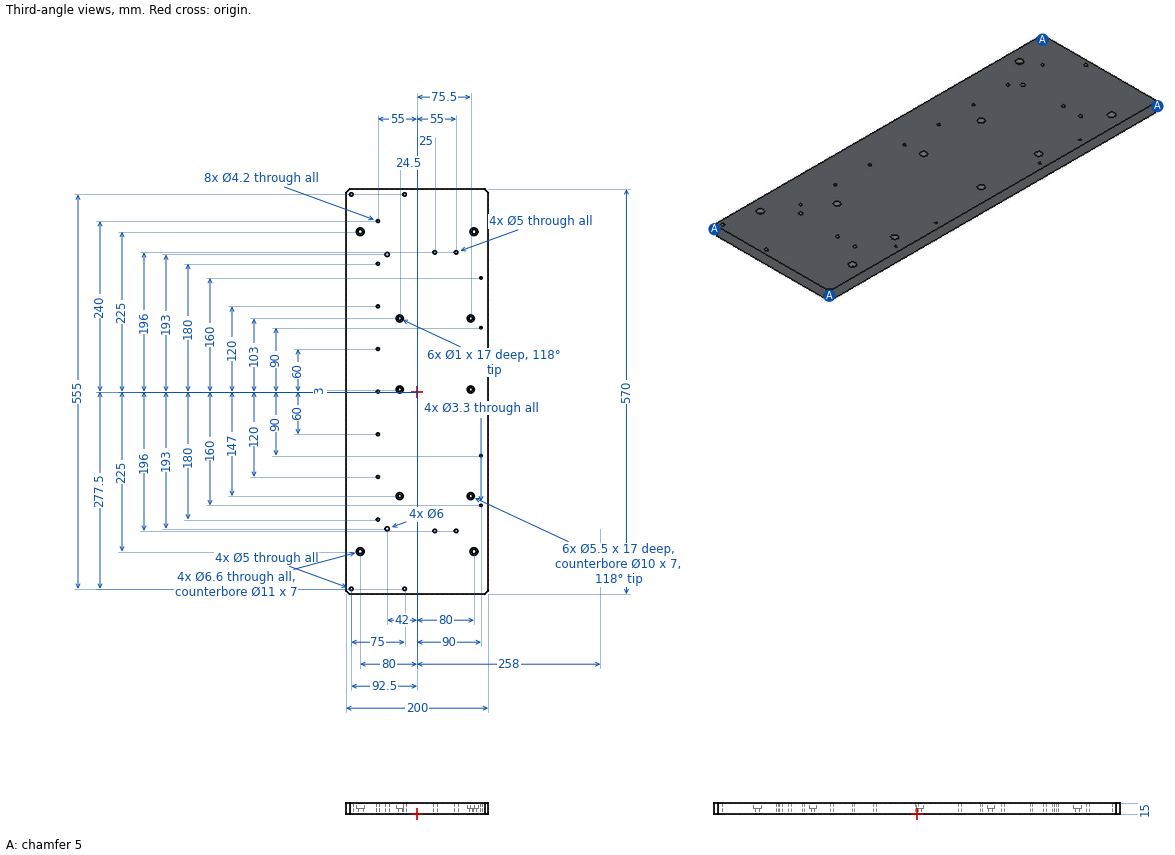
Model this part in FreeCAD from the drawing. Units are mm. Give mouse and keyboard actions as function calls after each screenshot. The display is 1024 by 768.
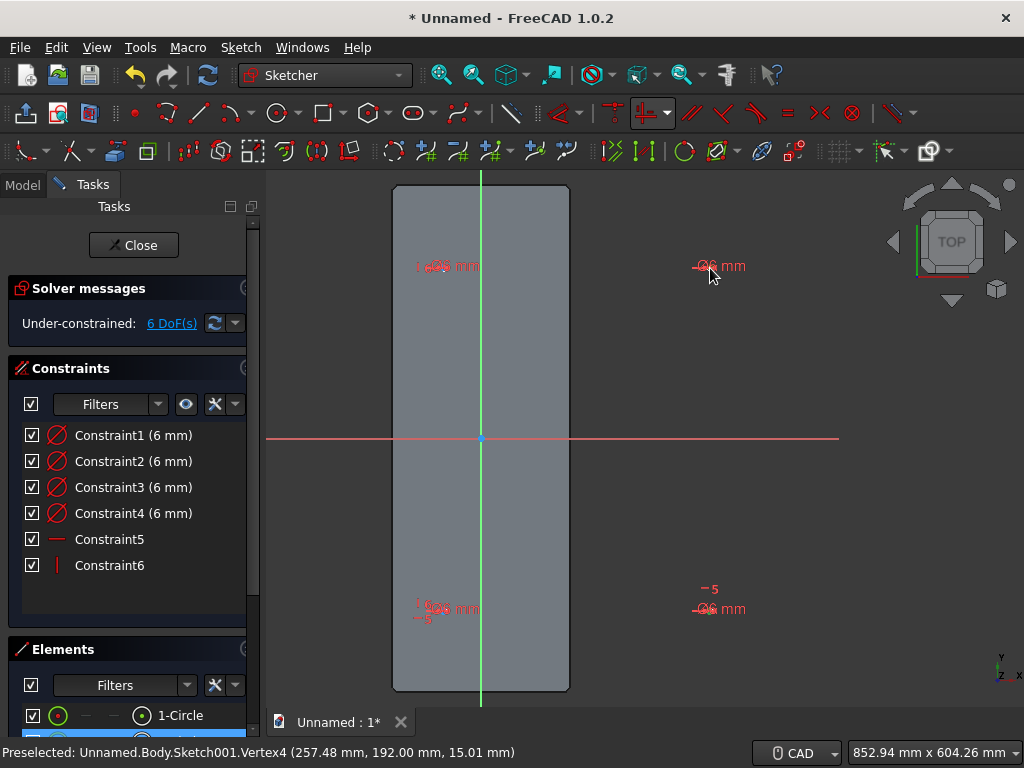
click(670, 114)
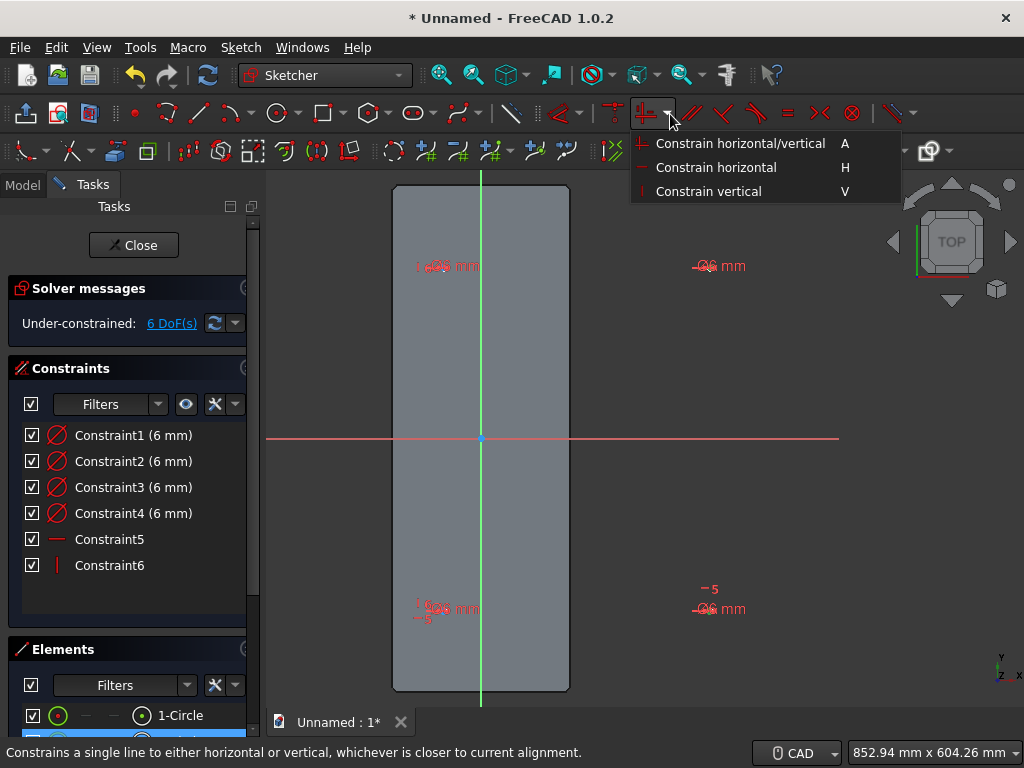
click(766, 191)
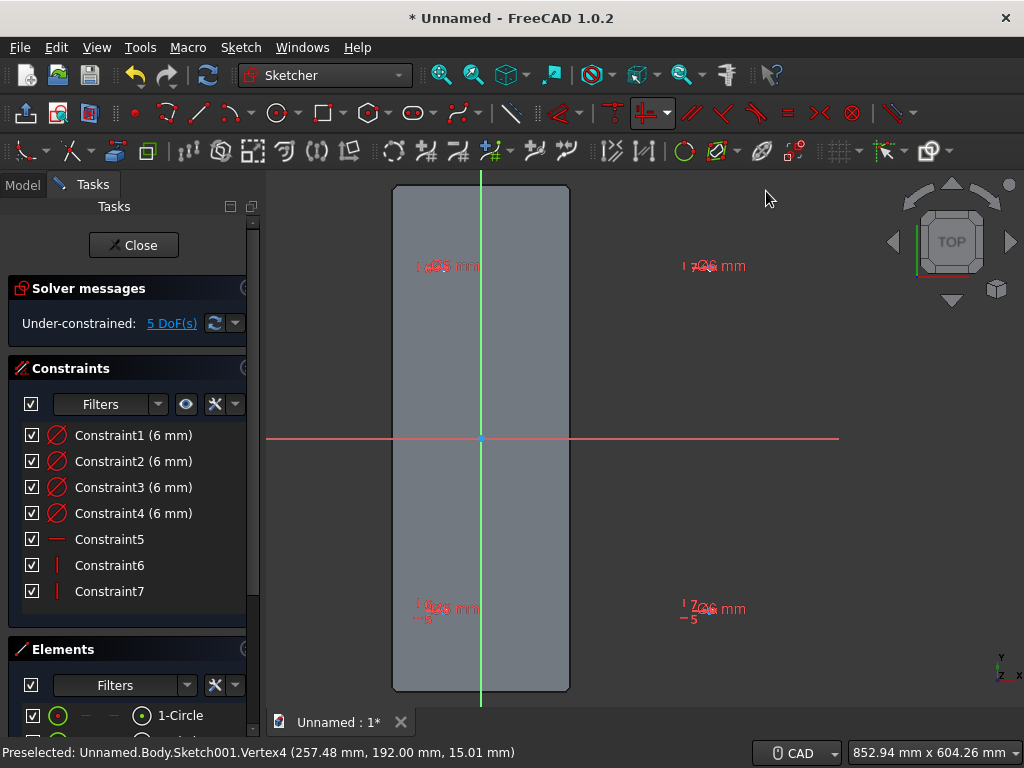
click(444, 268)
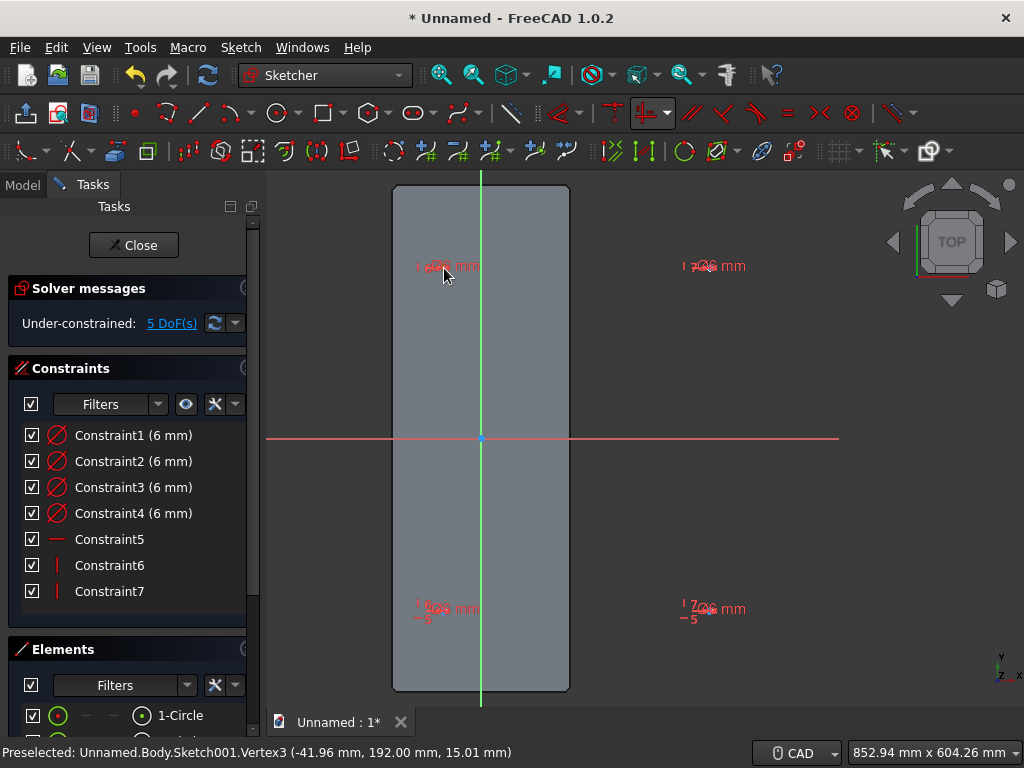
click(710, 268)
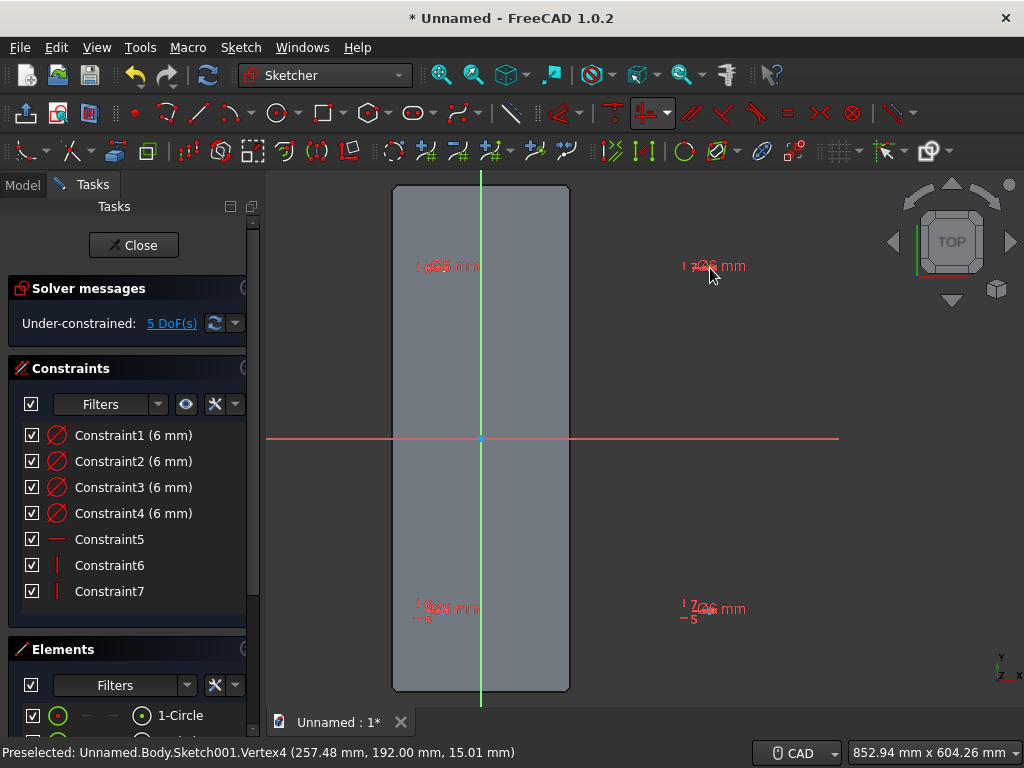
click(670, 114)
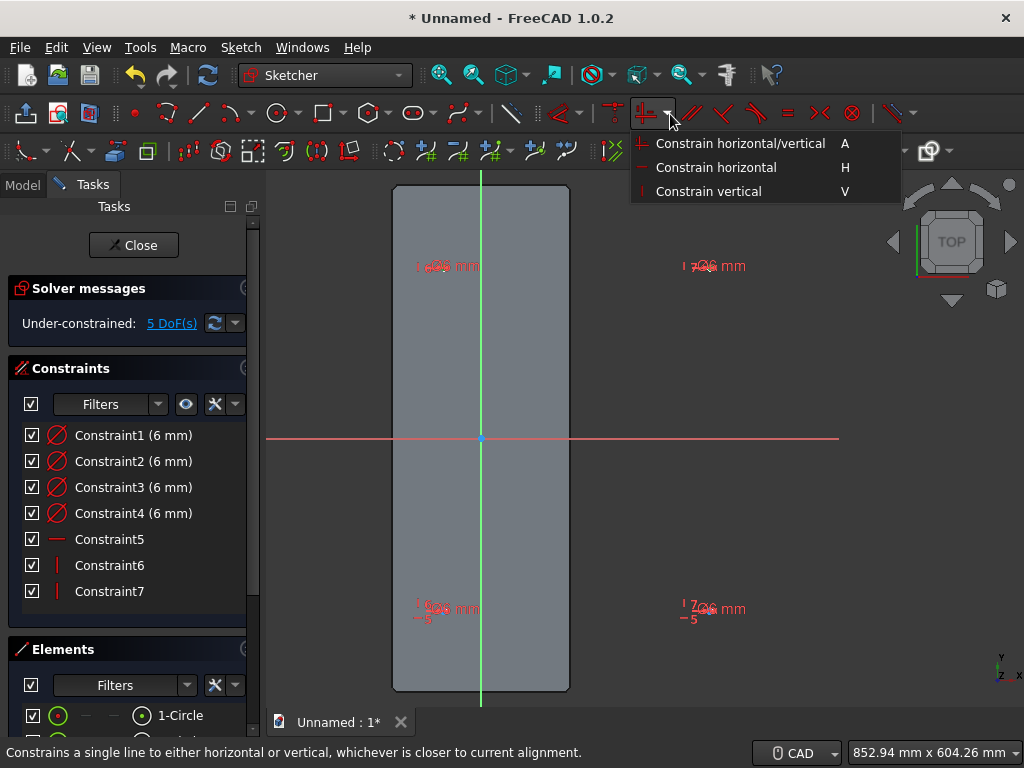
click(766, 167)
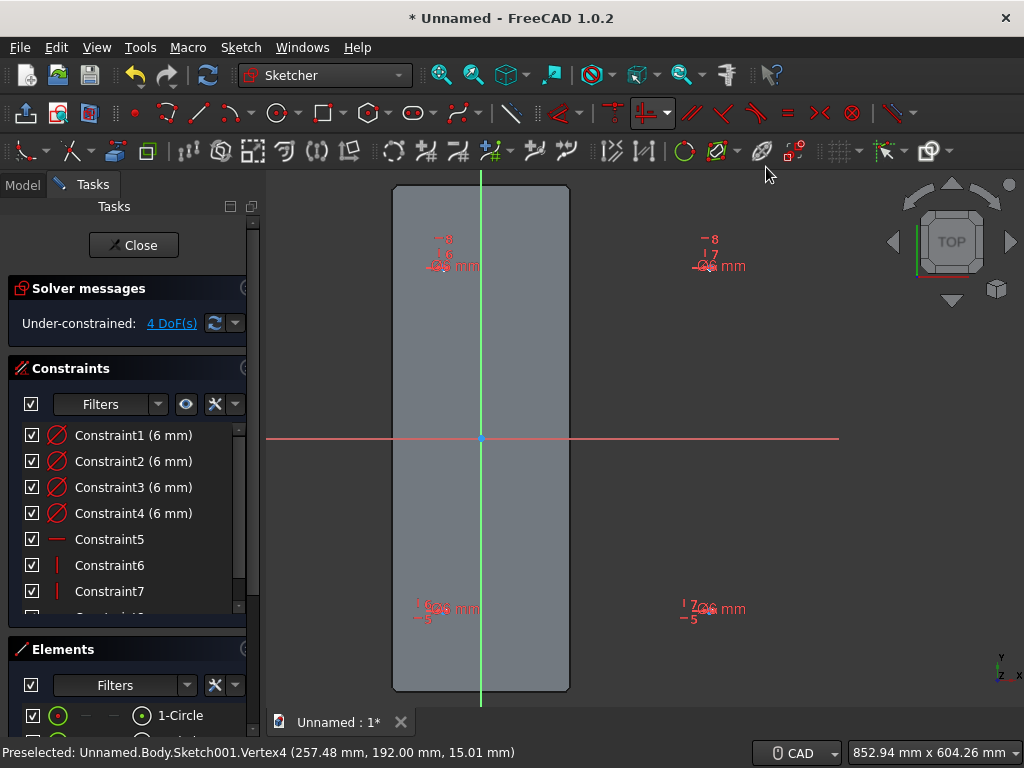
click(558, 114)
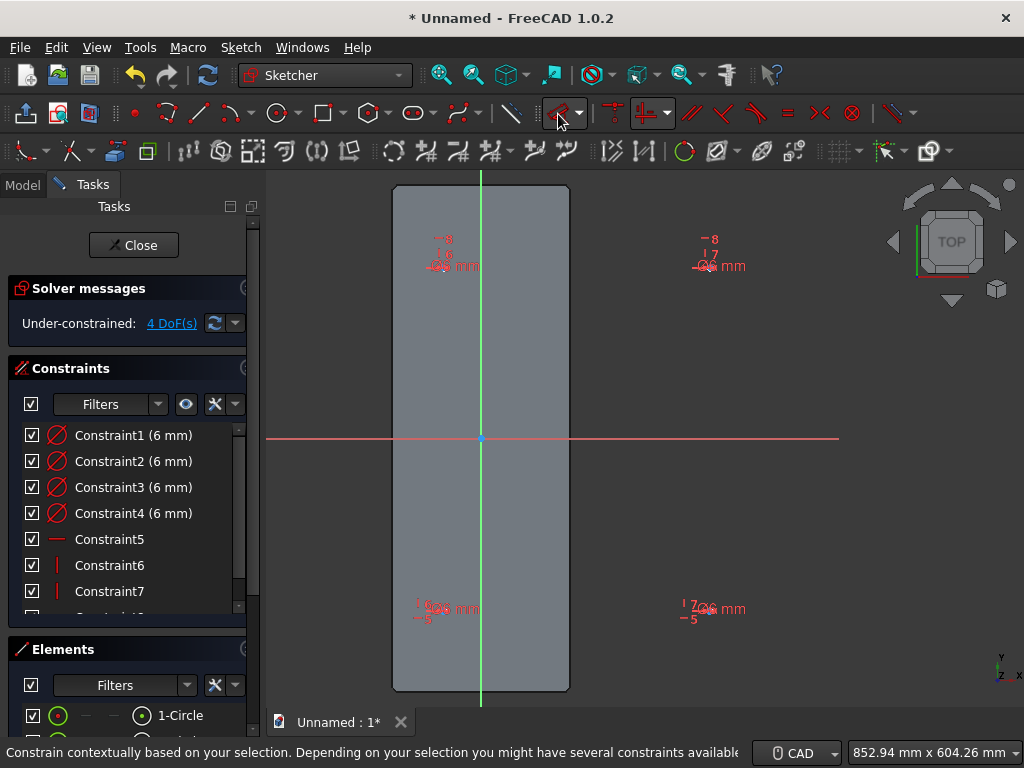
click(444, 611)
click(463, 645)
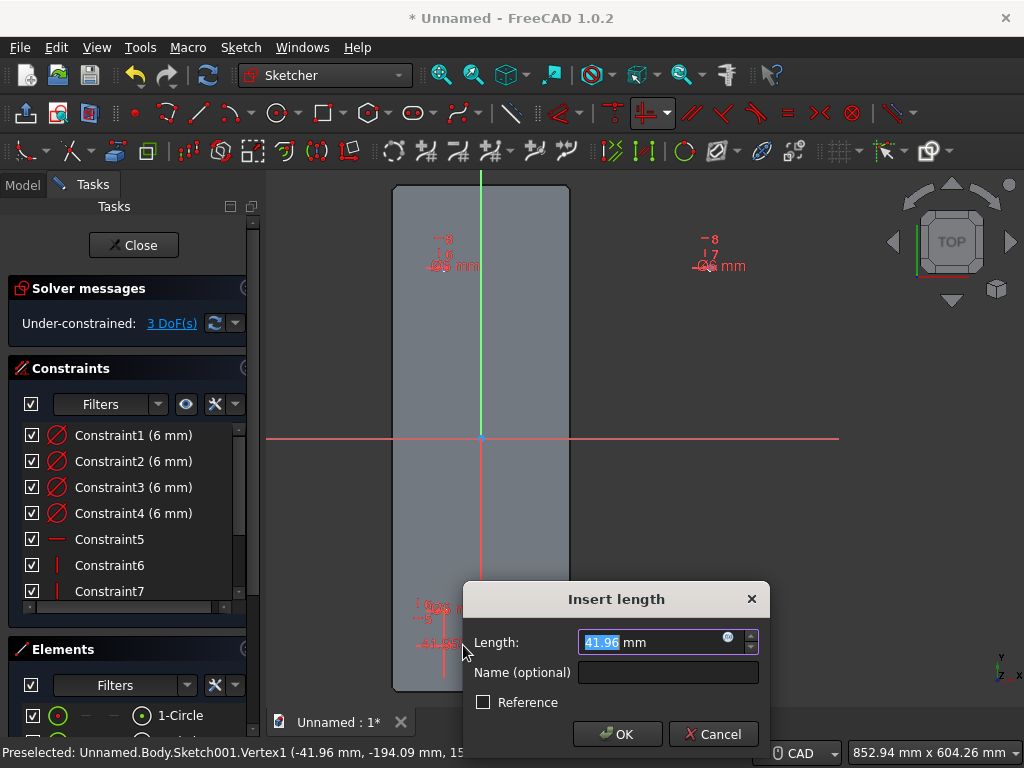
text(42)
key(Return)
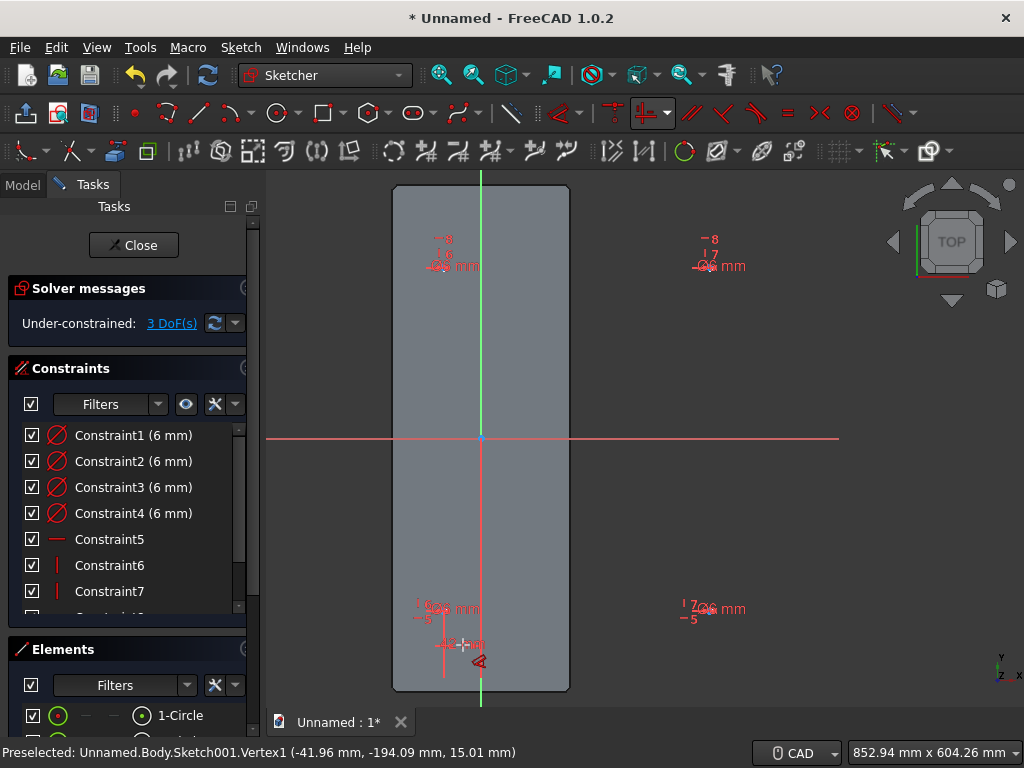
click(444, 611)
click(410, 525)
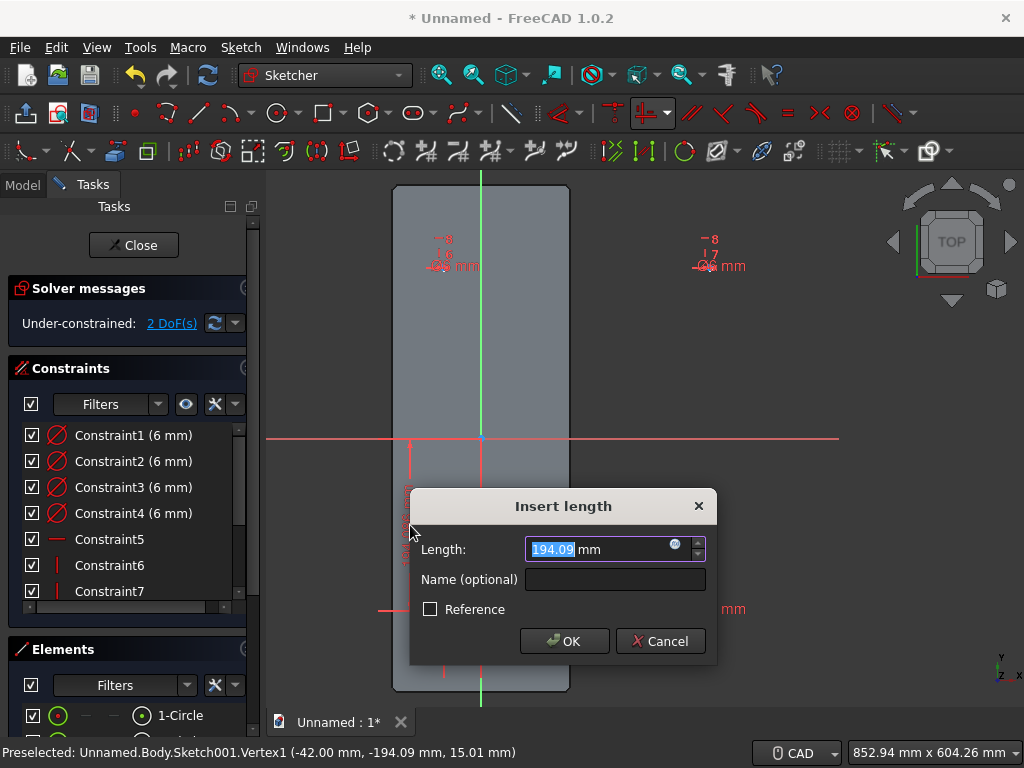
text(193)
key(Return)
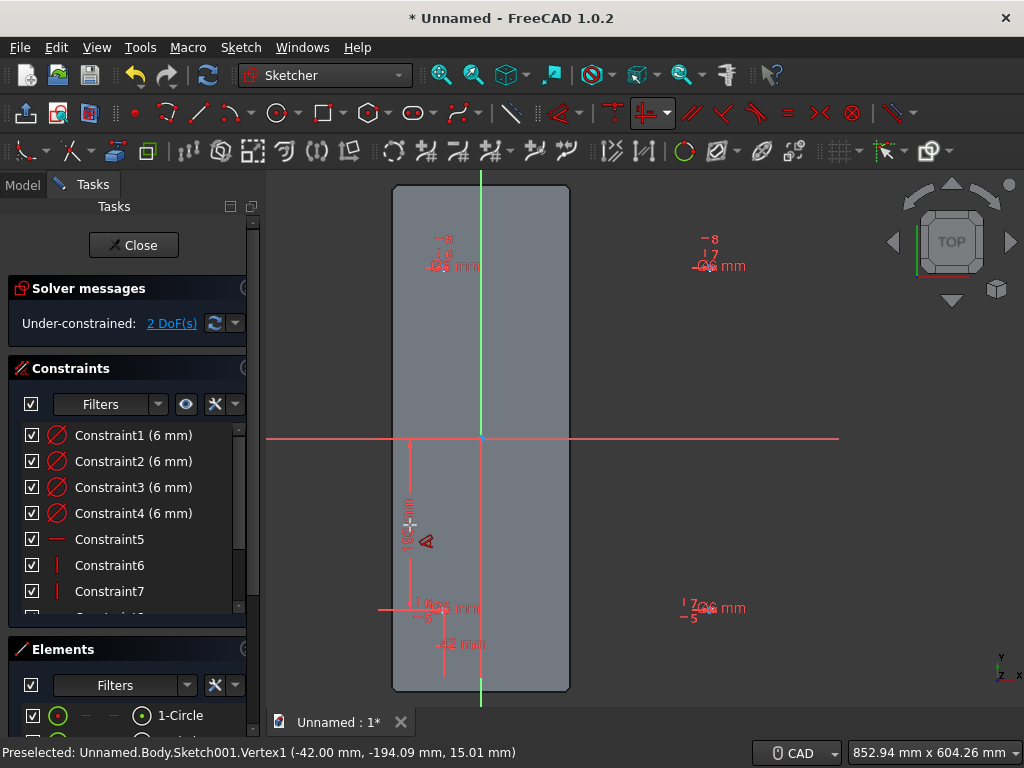
click(710, 610)
click(596, 644)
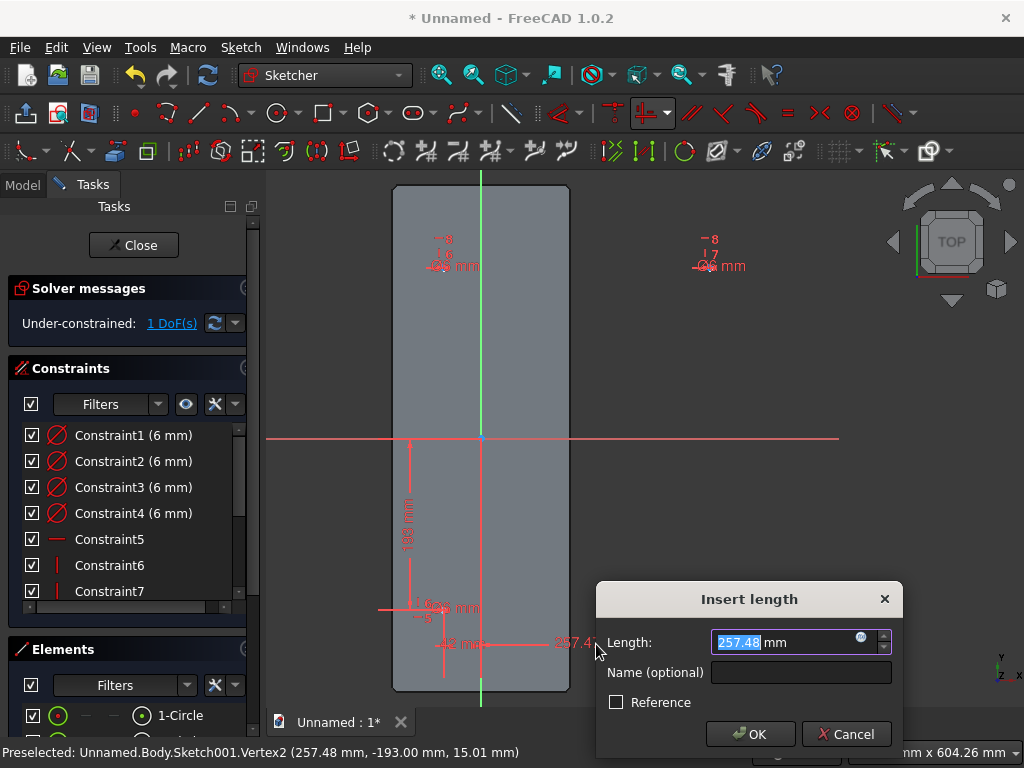
text(258)
key(Return)